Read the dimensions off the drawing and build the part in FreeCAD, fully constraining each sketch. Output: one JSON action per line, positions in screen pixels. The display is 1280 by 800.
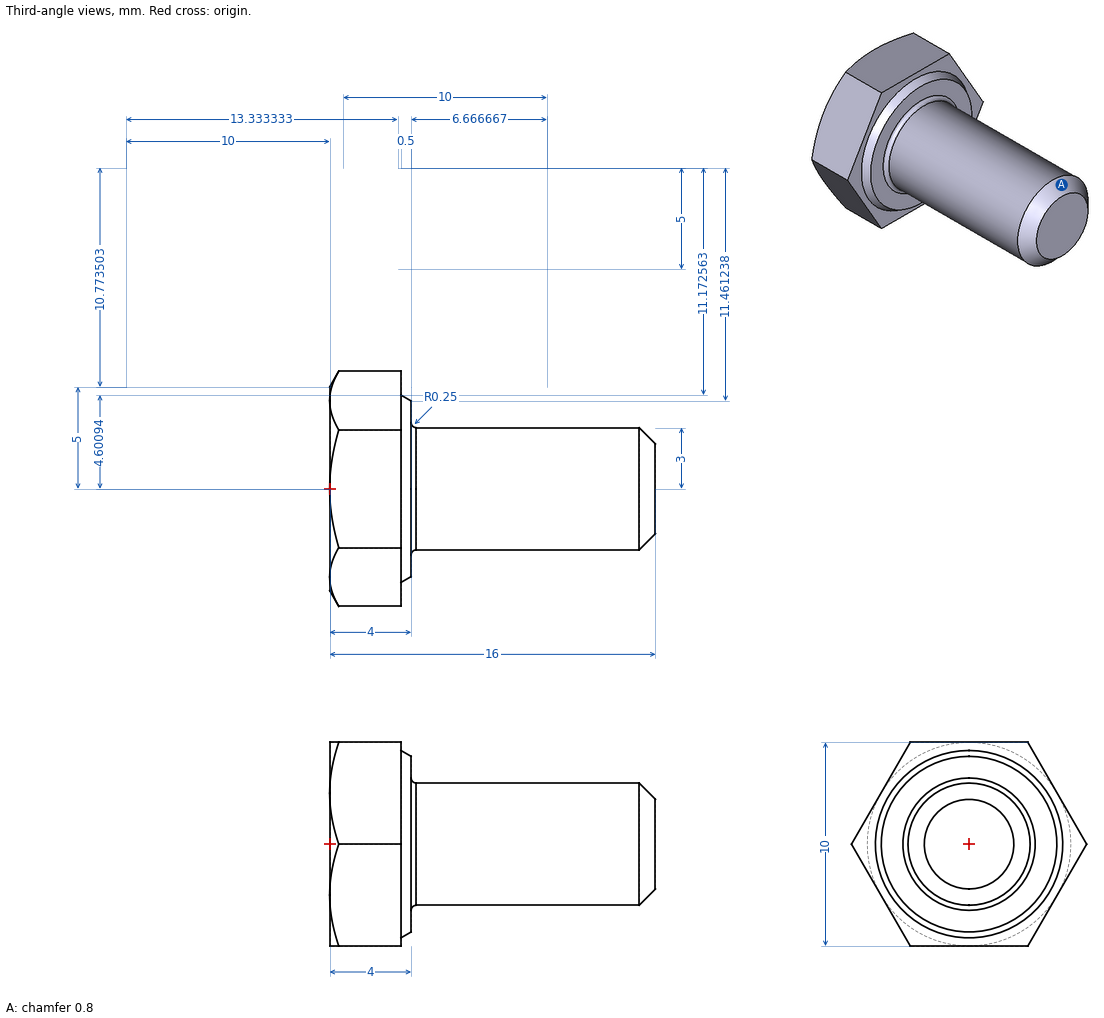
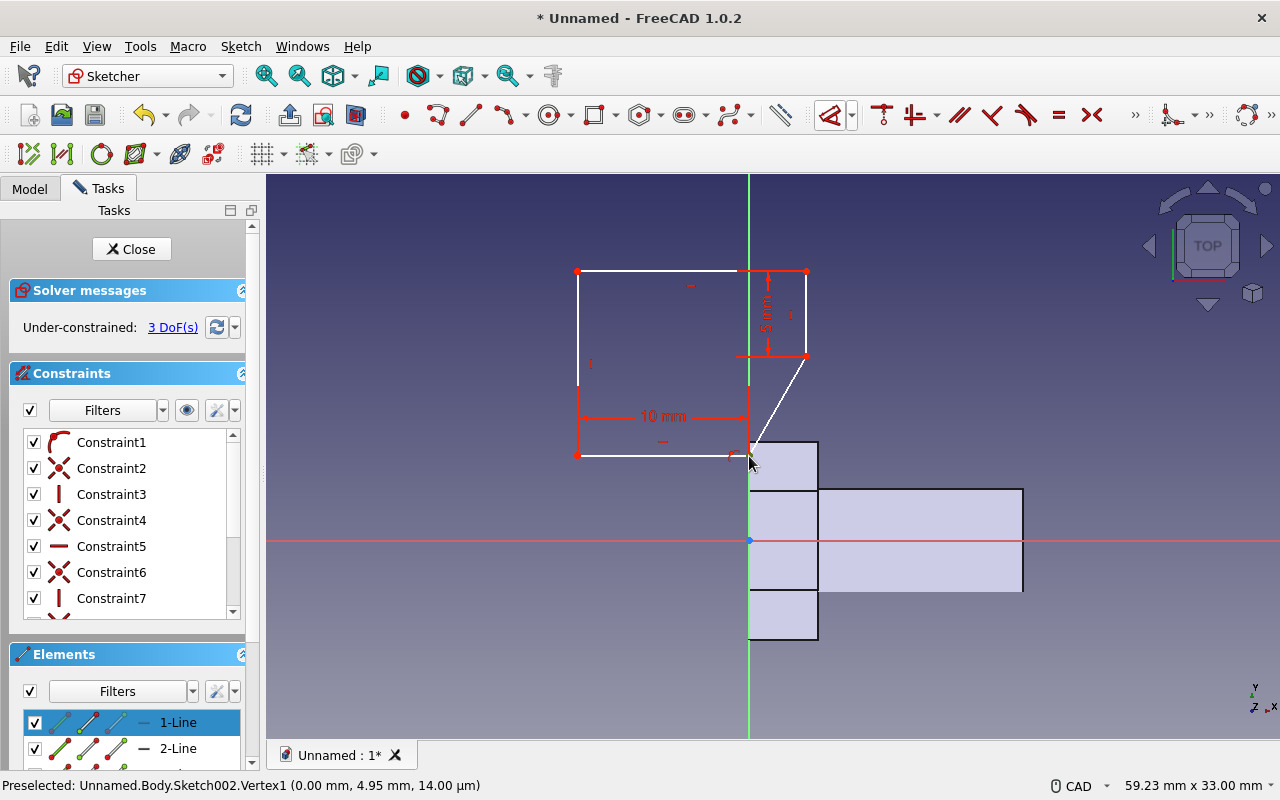
{"action": "left_click", "coordinate": [852, 116]}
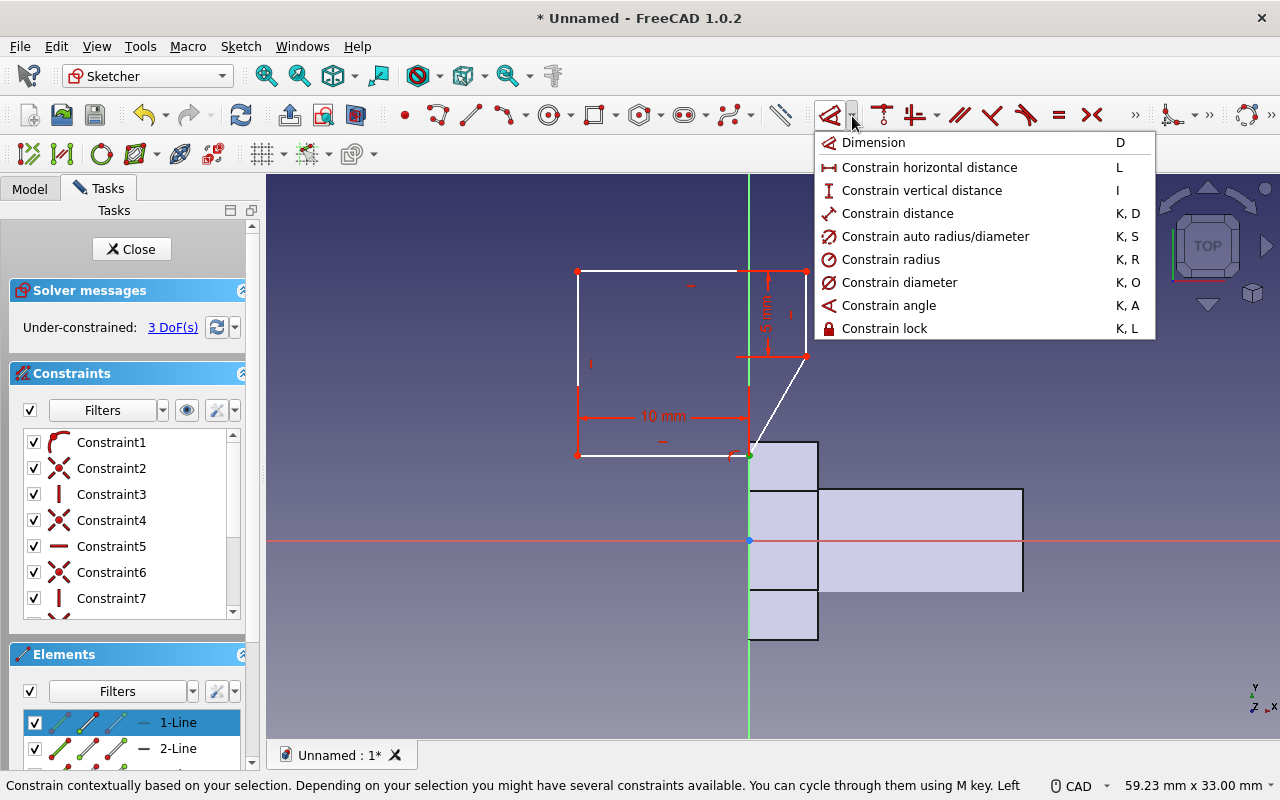
{"action": "left_click", "coordinate": [985, 190]}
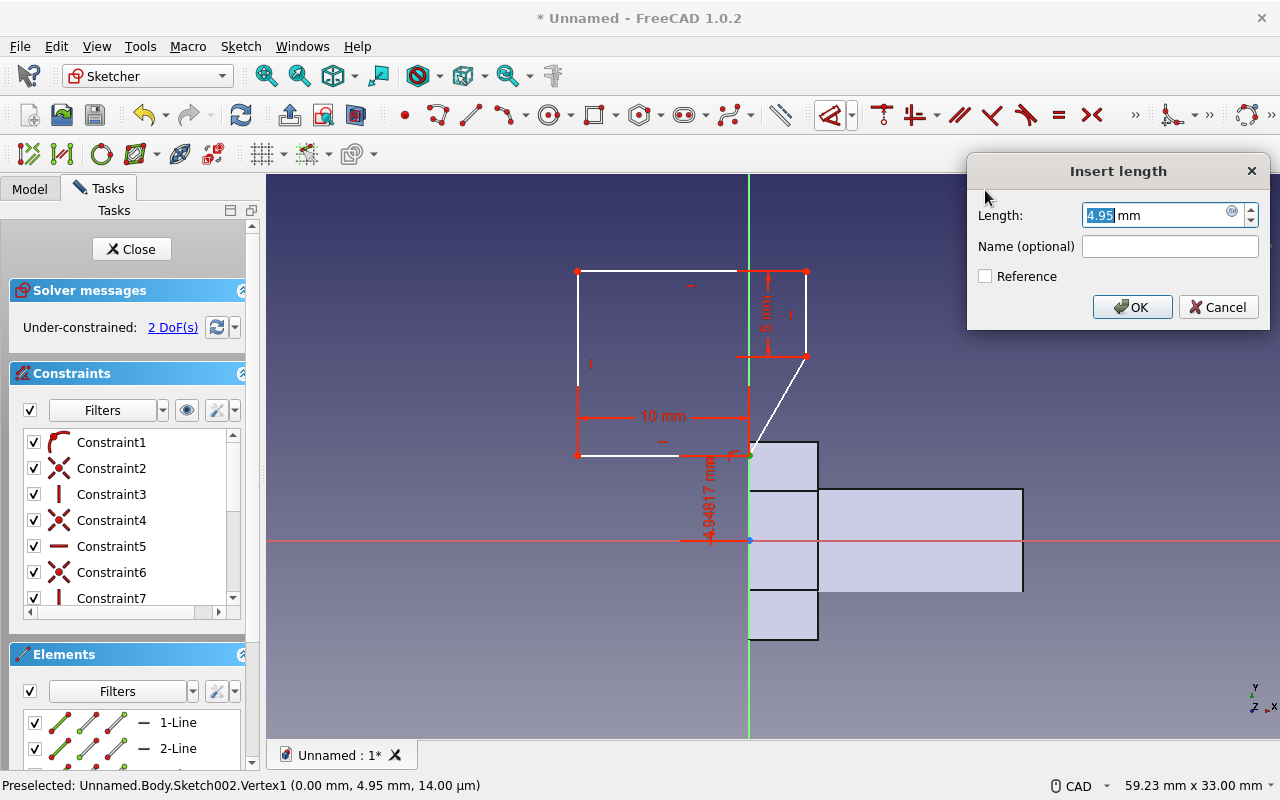
{"action": "type", "text": "5"}
{"action": "key", "text": "Return"}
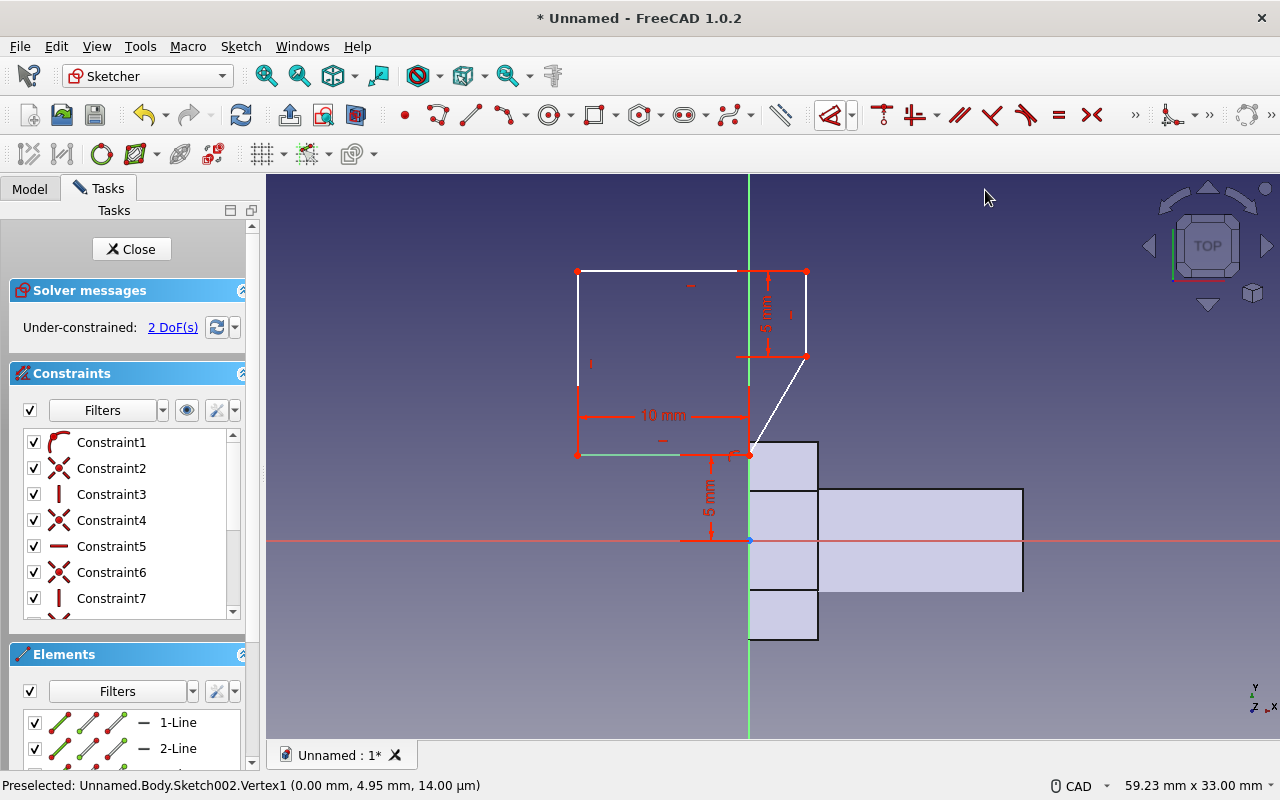
{"action": "left_click", "coordinate": [738, 271]}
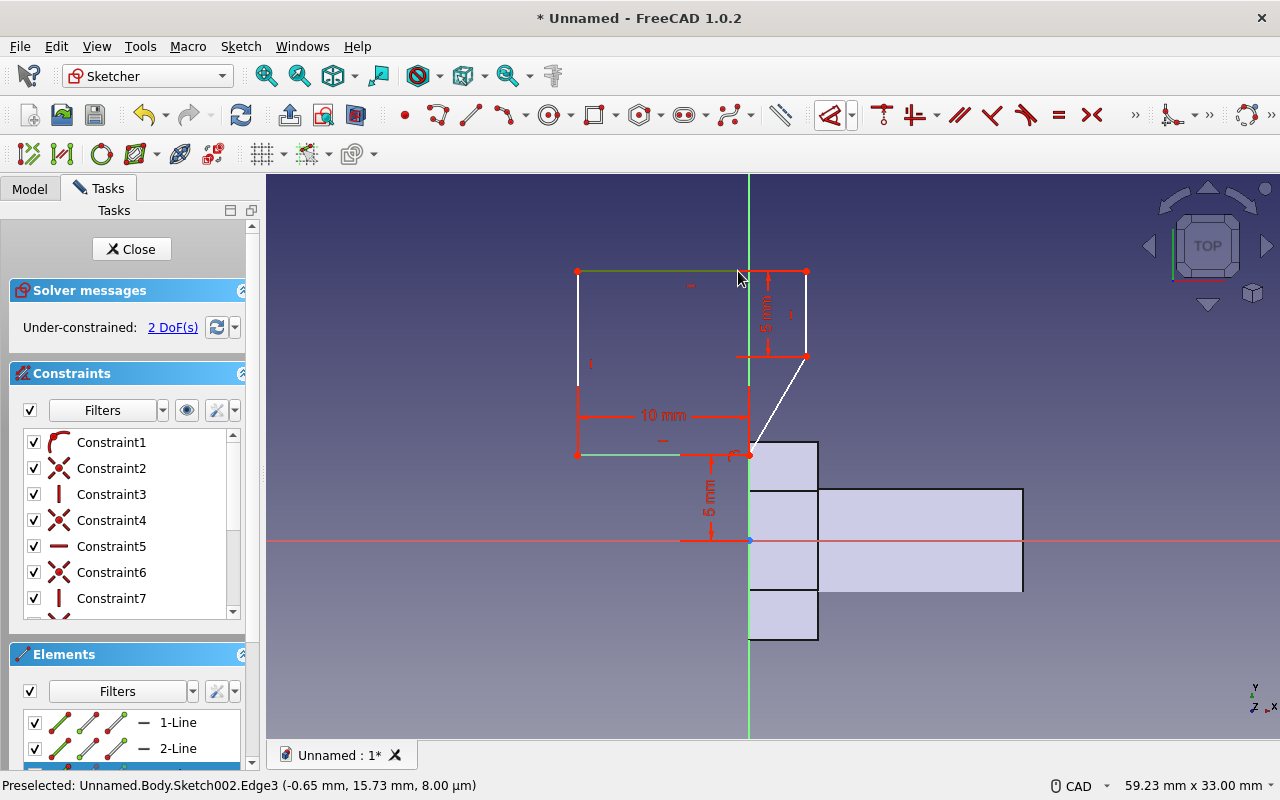
{"action": "left_click", "coordinate": [852, 116]}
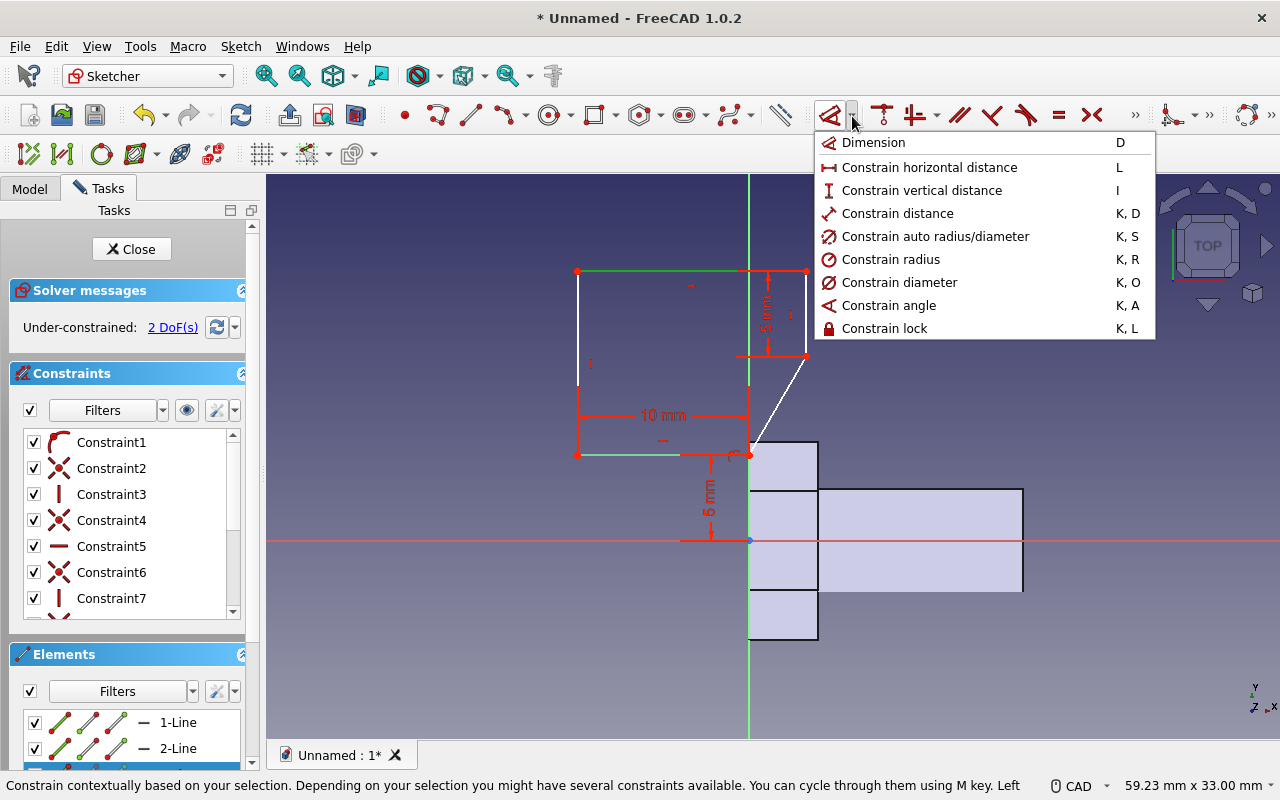
{"action": "left_click", "coordinate": [985, 168]}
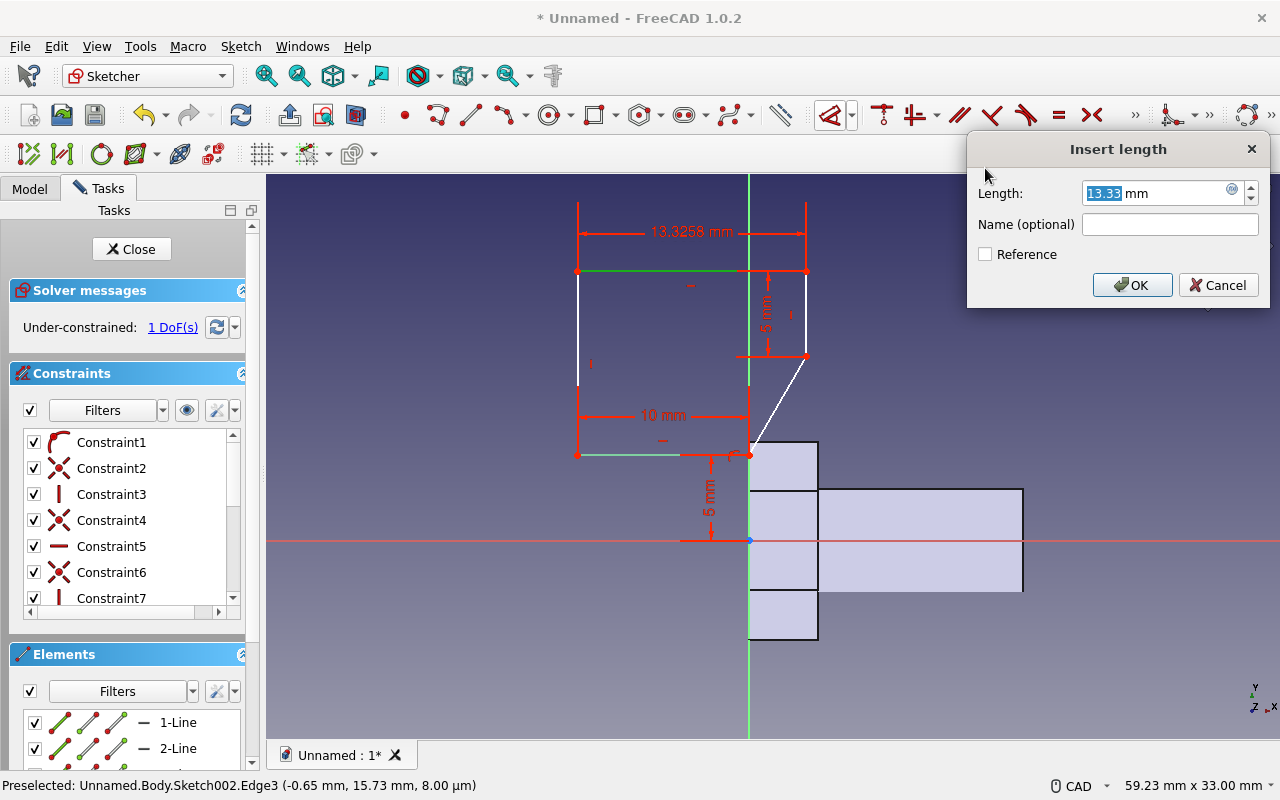
{"action": "type", "text": "13.333333"}
{"action": "key", "text": "Return"}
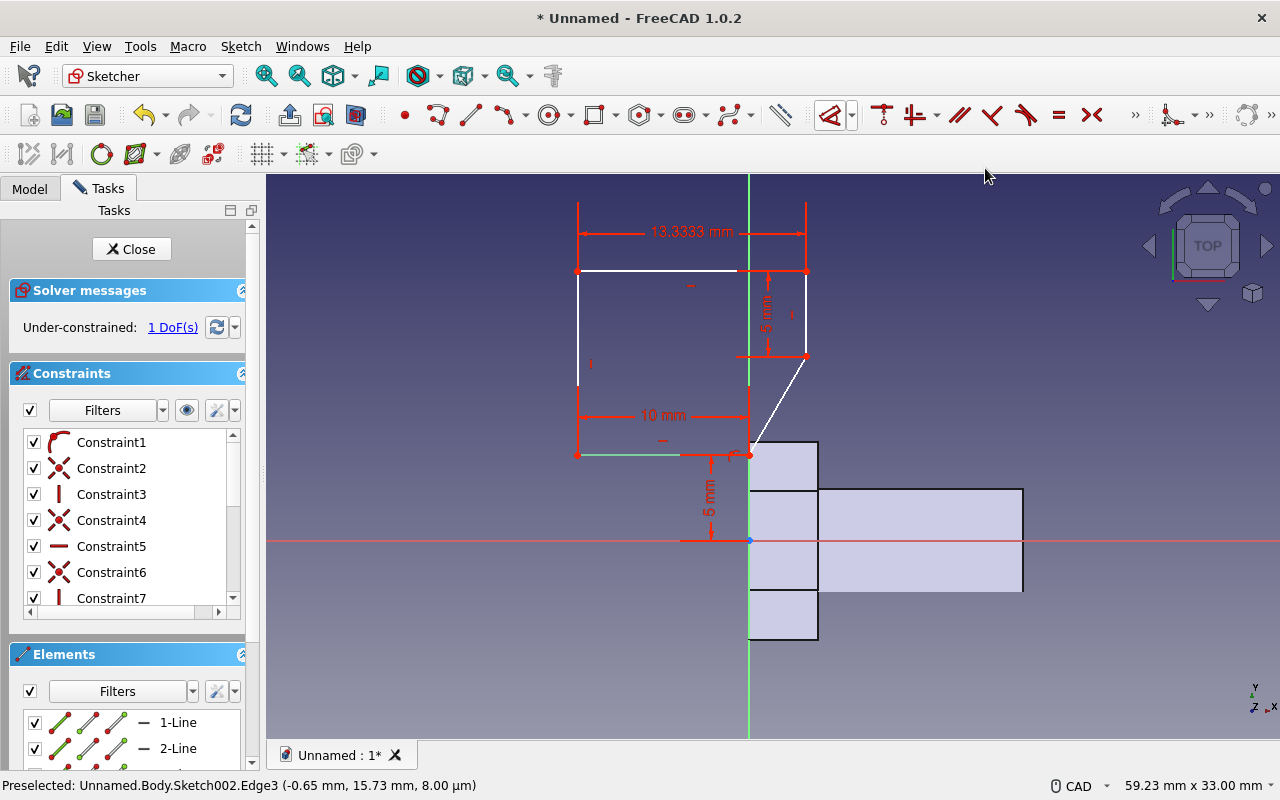
{"action": "left_click", "coordinate": [578, 327]}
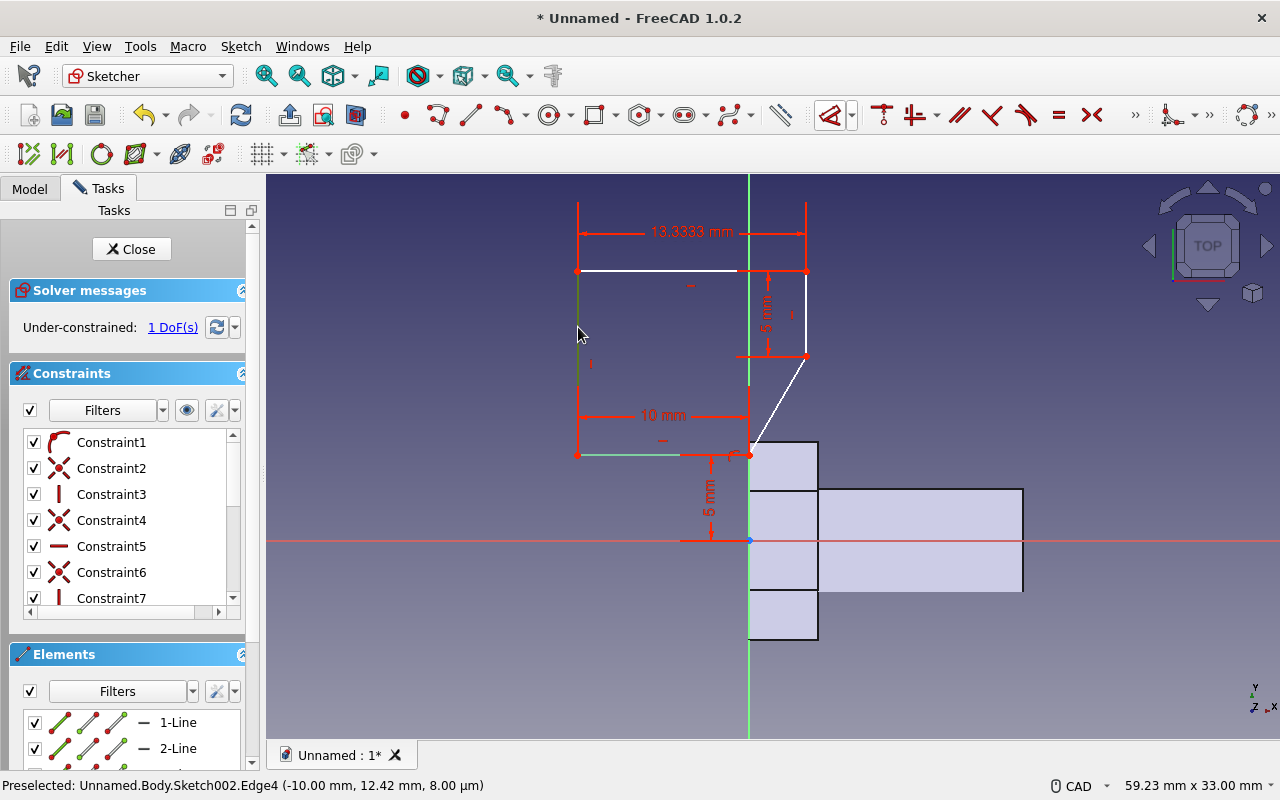
{"action": "left_click", "coordinate": [852, 116]}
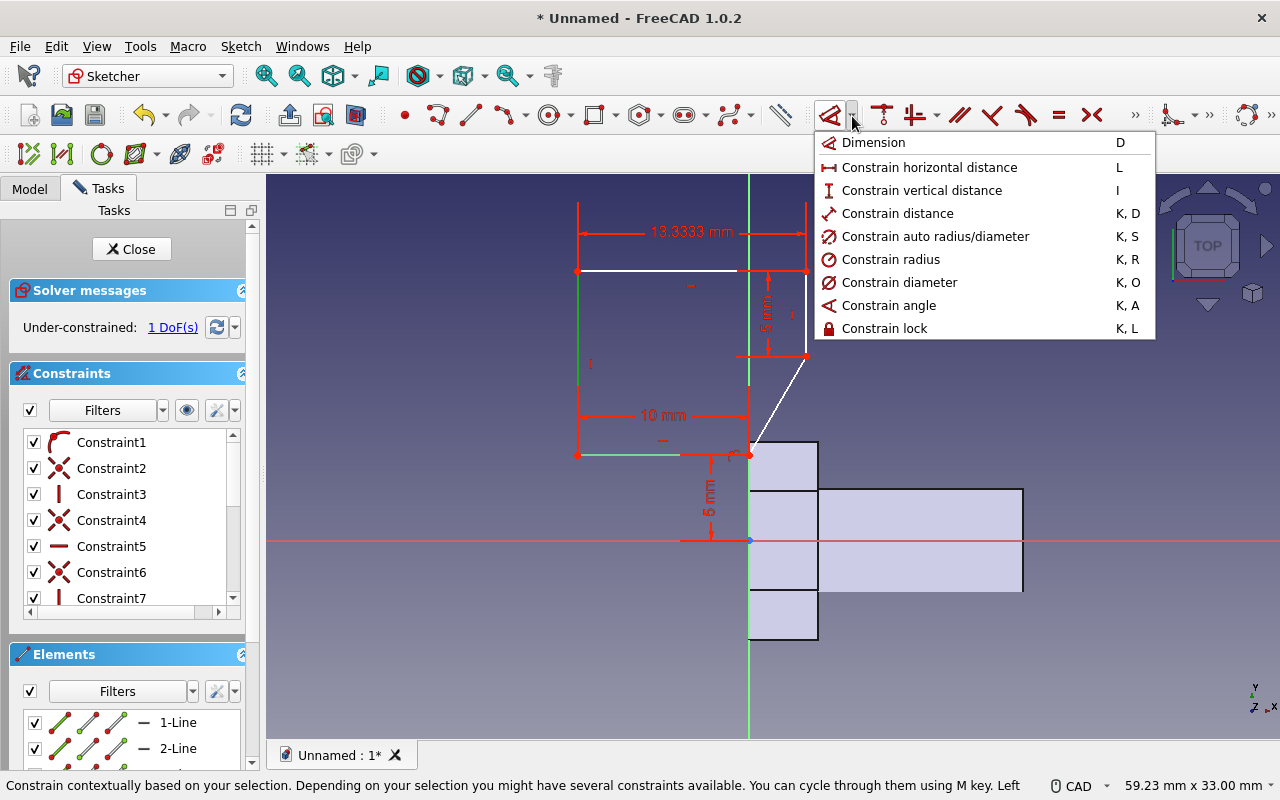
{"action": "left_click", "coordinate": [985, 190]}